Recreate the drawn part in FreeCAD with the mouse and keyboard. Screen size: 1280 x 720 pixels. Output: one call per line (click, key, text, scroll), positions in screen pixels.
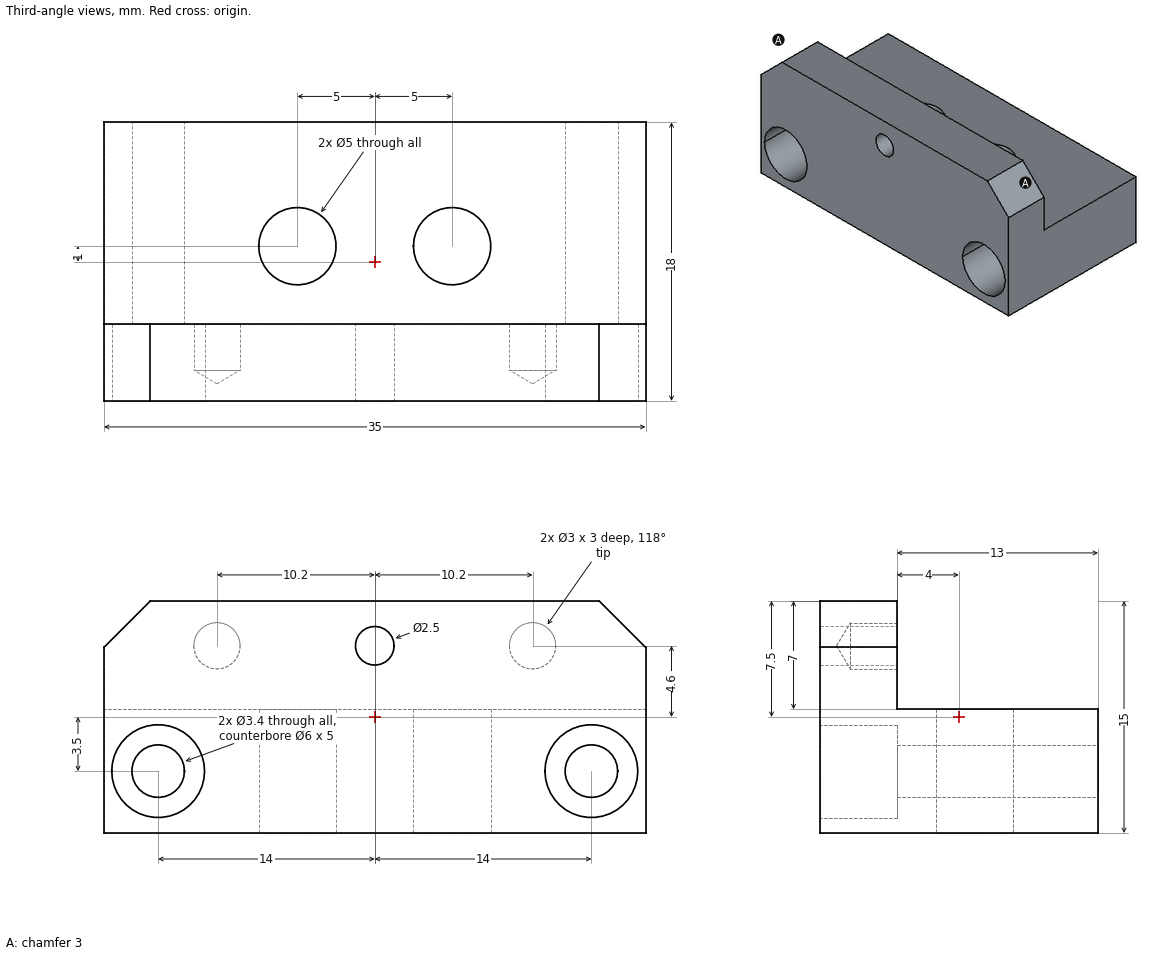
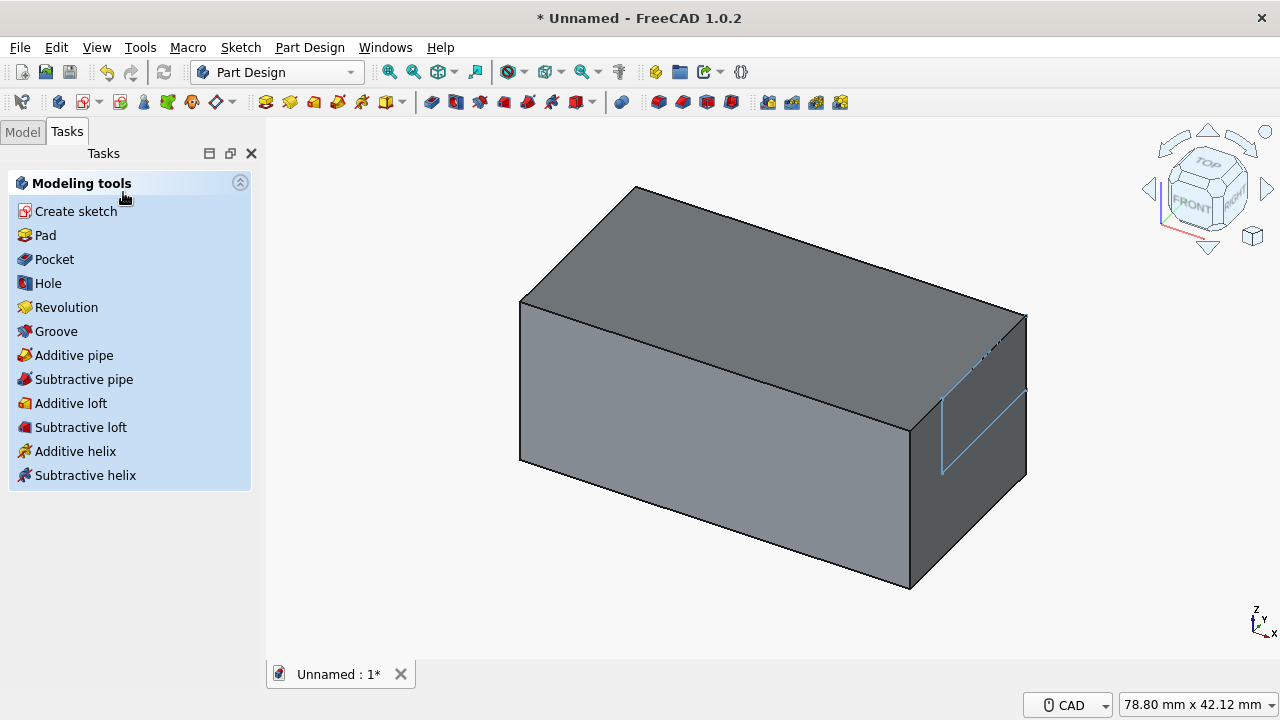
click(432, 102)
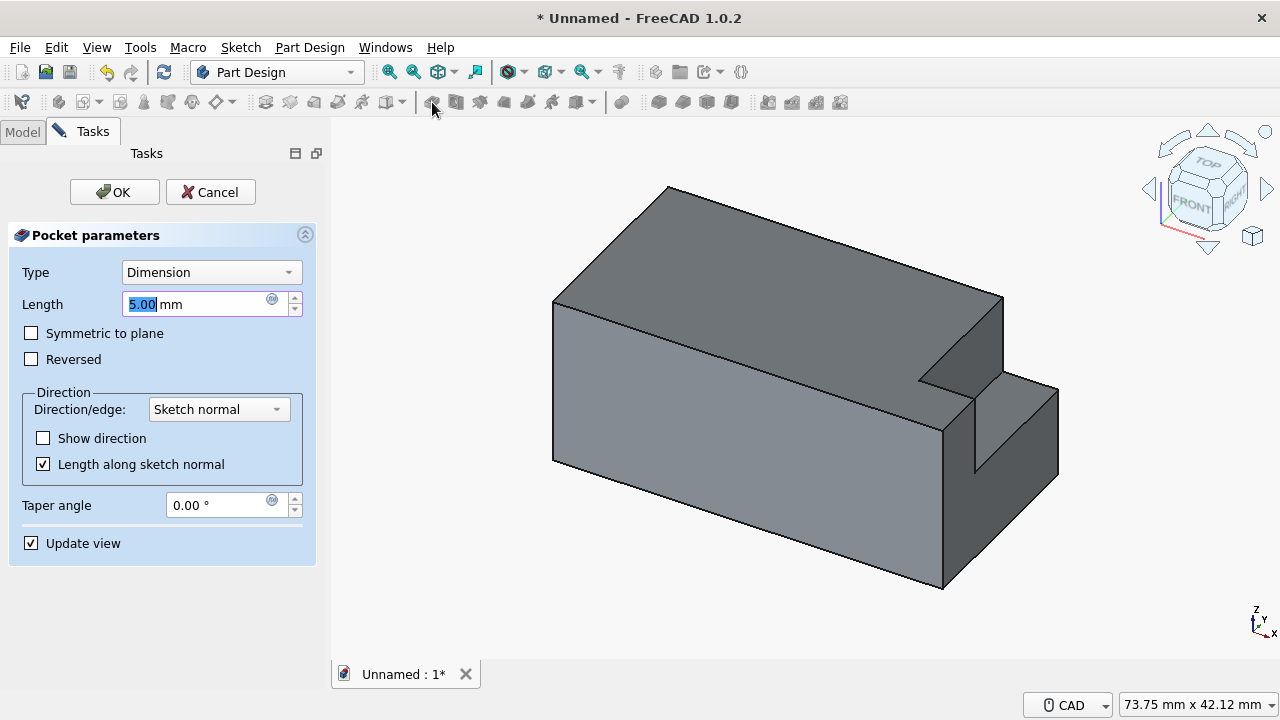
click(212, 272)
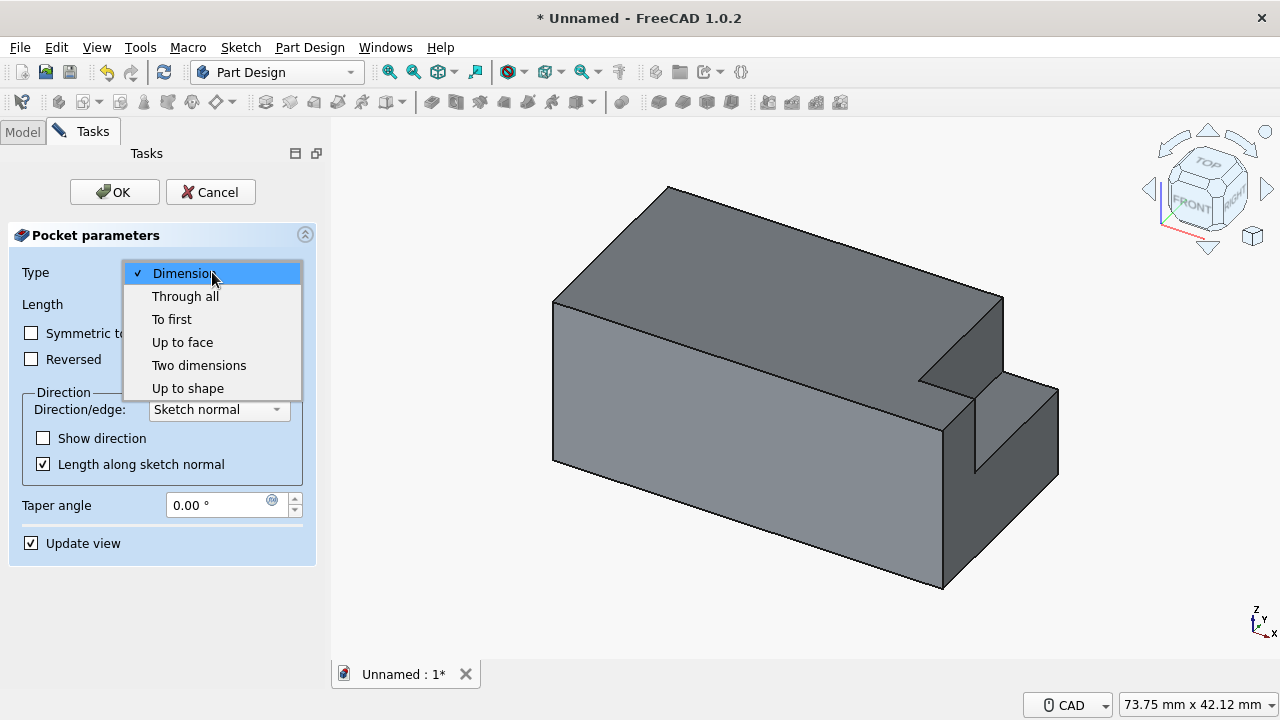
click(212, 296)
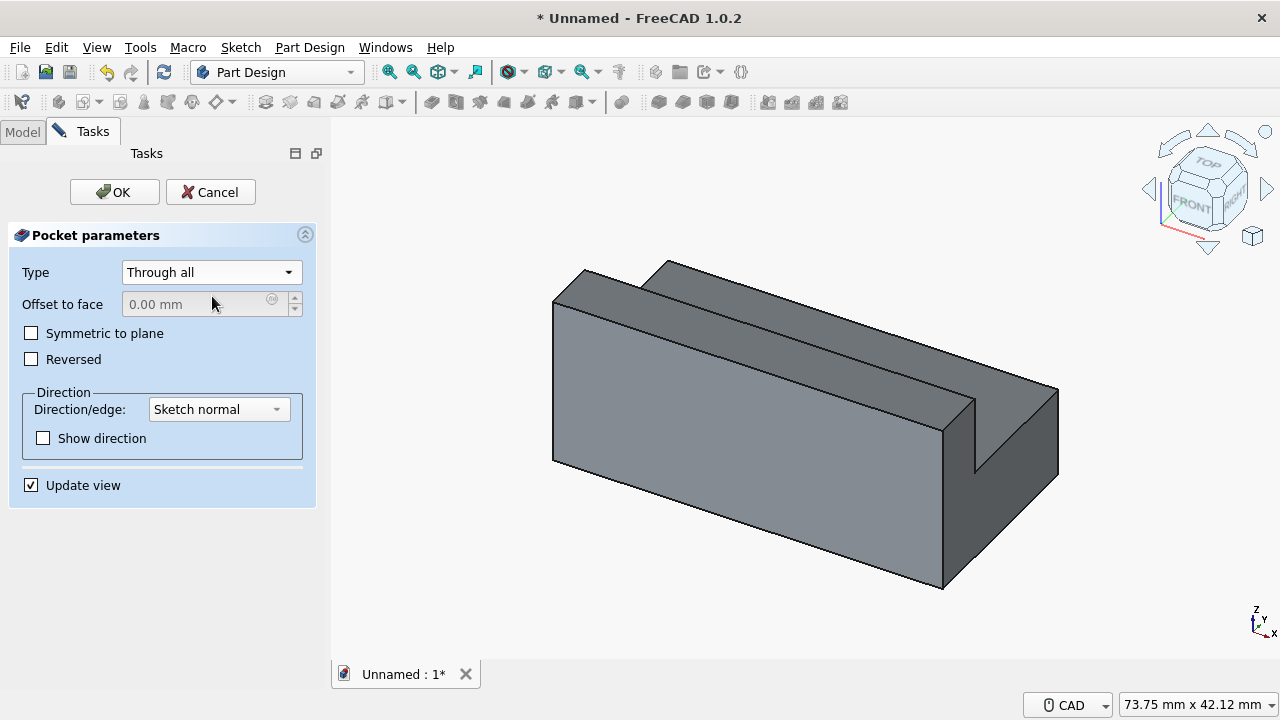
click(115, 192)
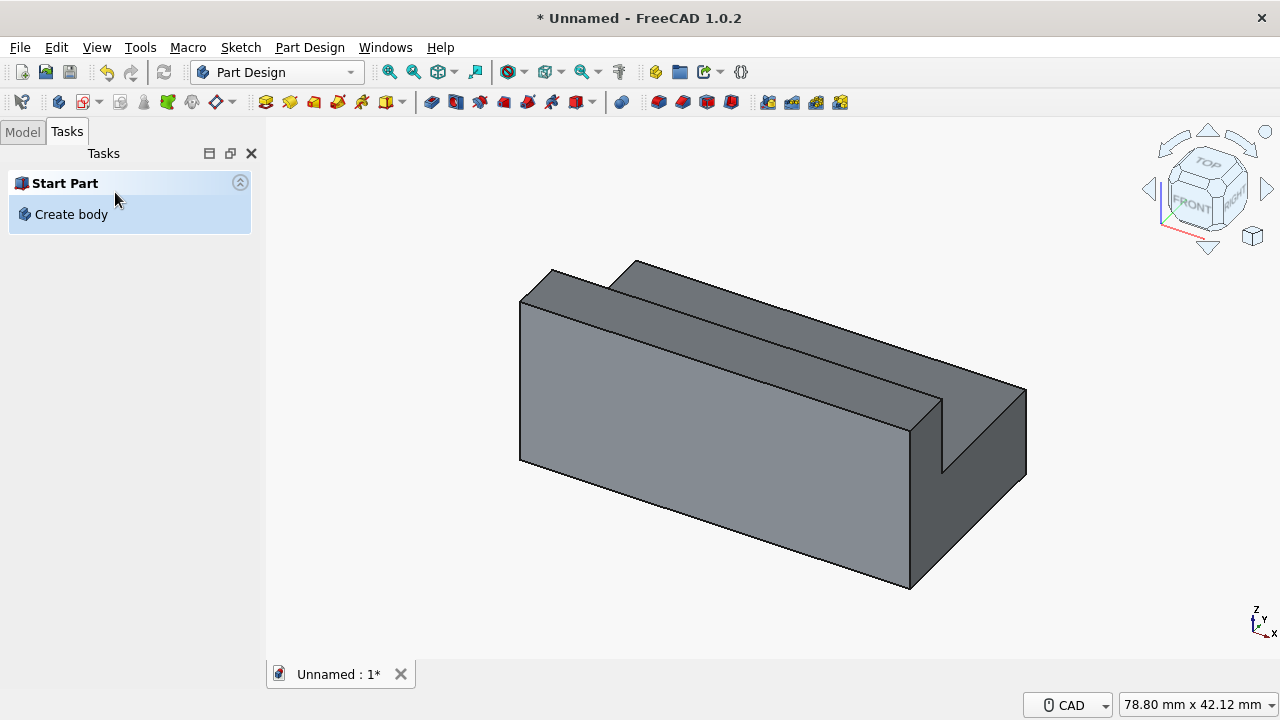
key(0)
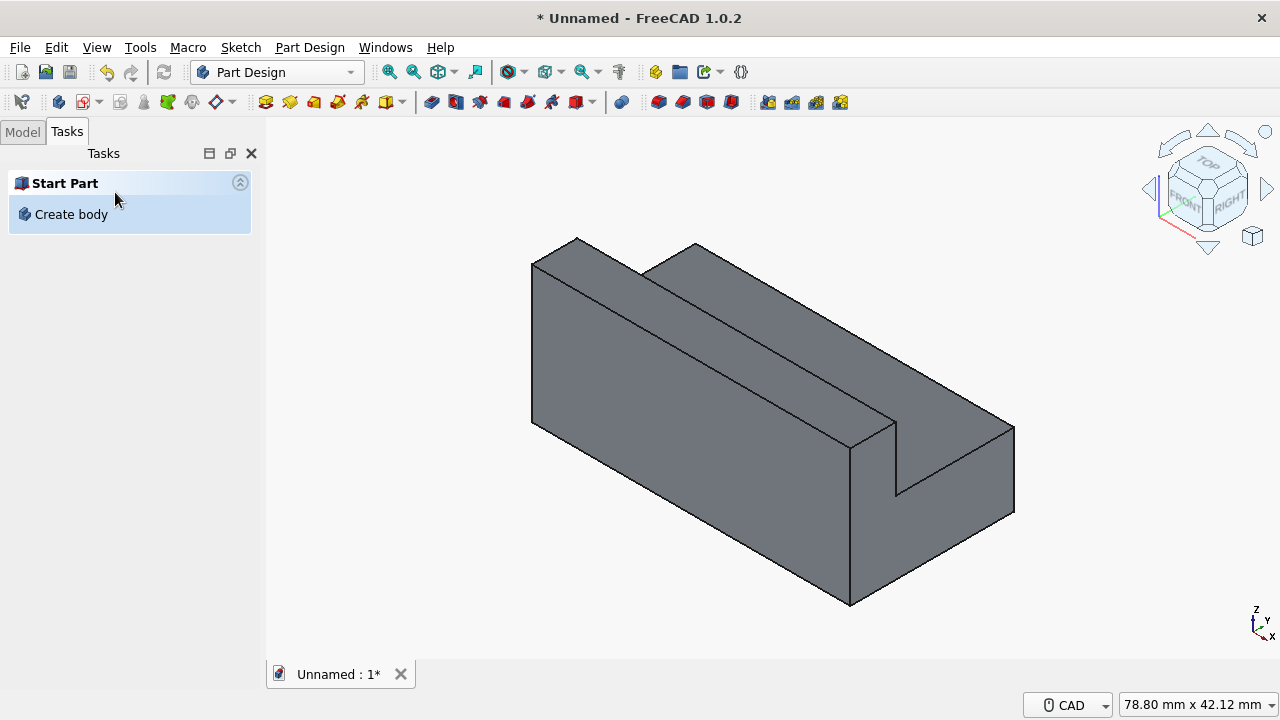
key(2)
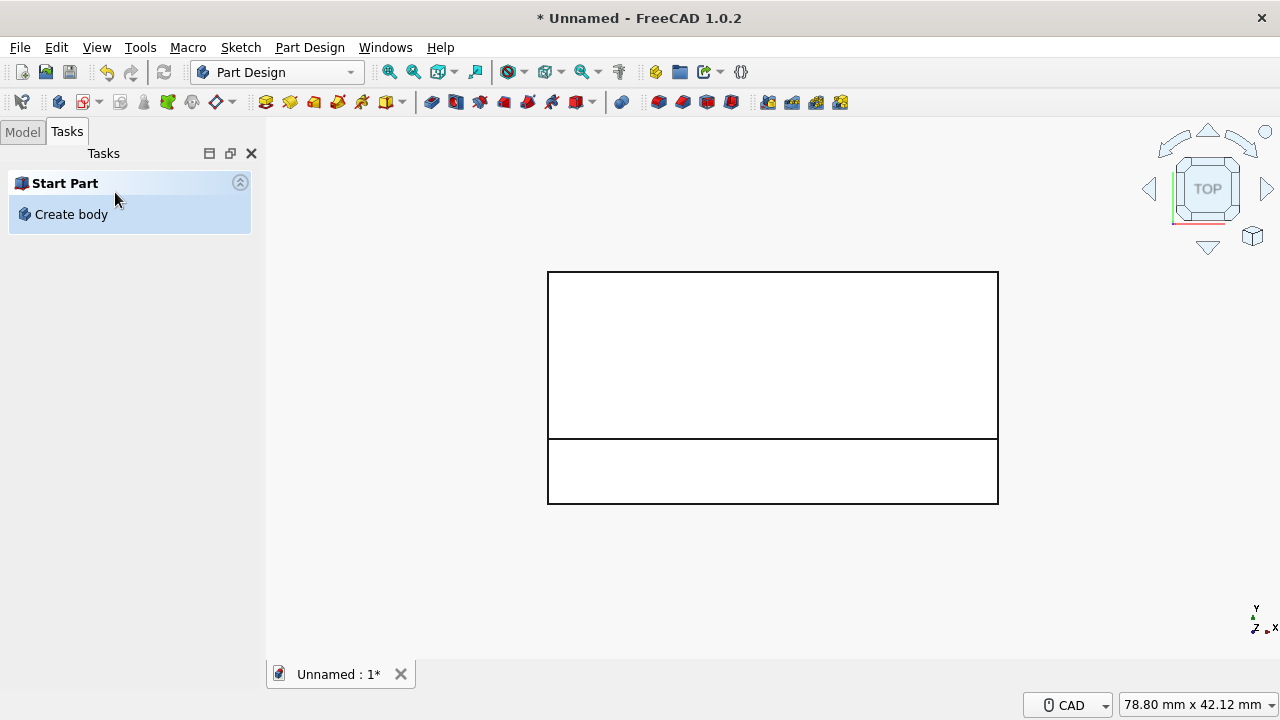
key(v)
key(f)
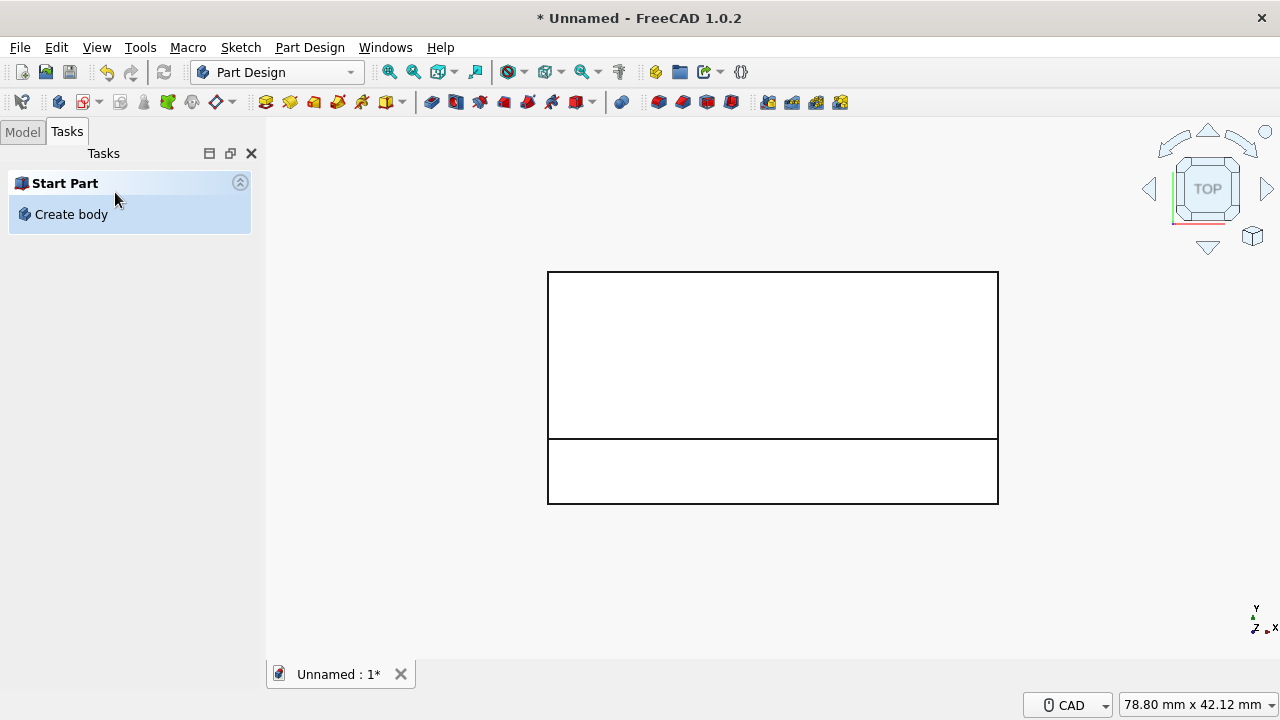
click(902, 355)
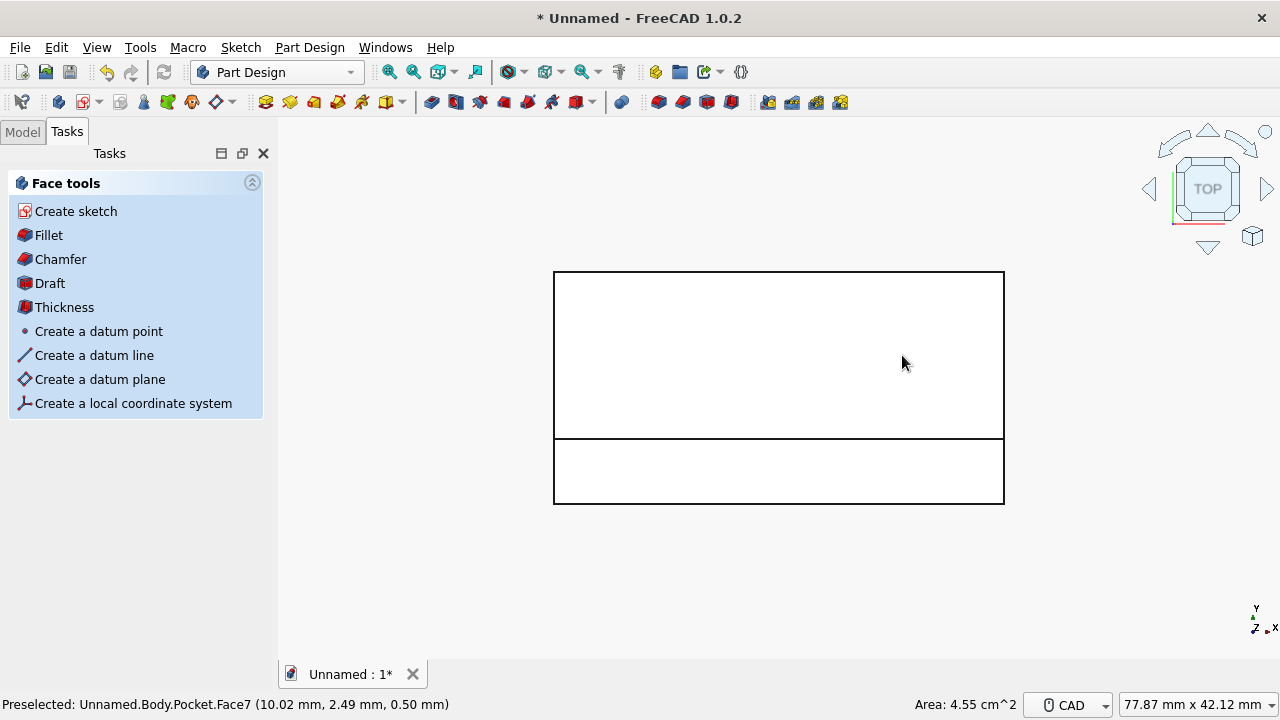
click(84, 102)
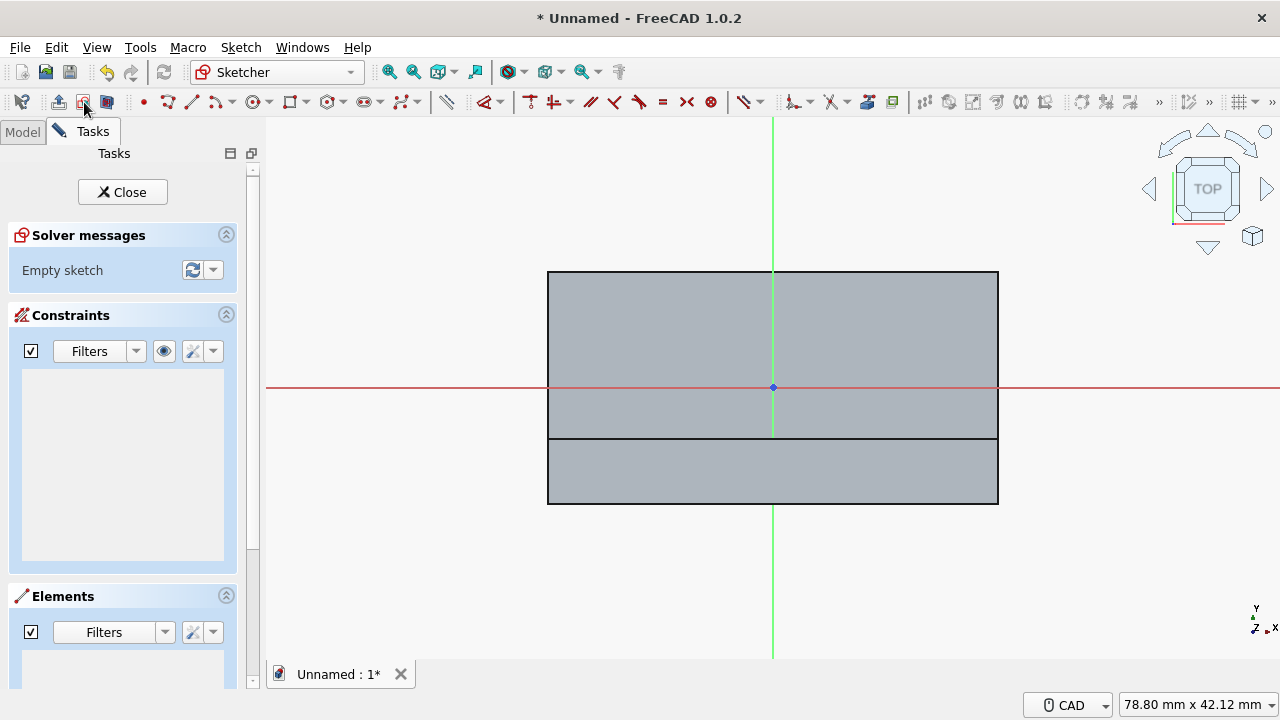
scroll(813, 368, up, 5)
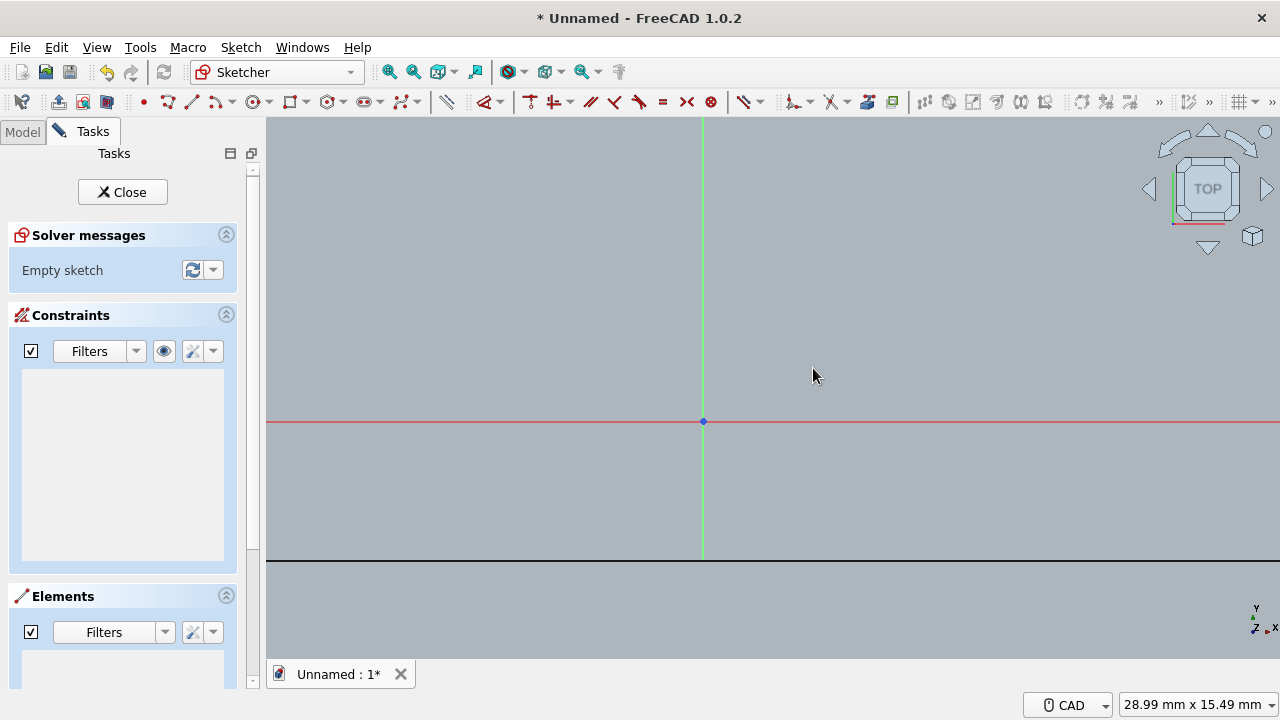
key(g)
key(c)